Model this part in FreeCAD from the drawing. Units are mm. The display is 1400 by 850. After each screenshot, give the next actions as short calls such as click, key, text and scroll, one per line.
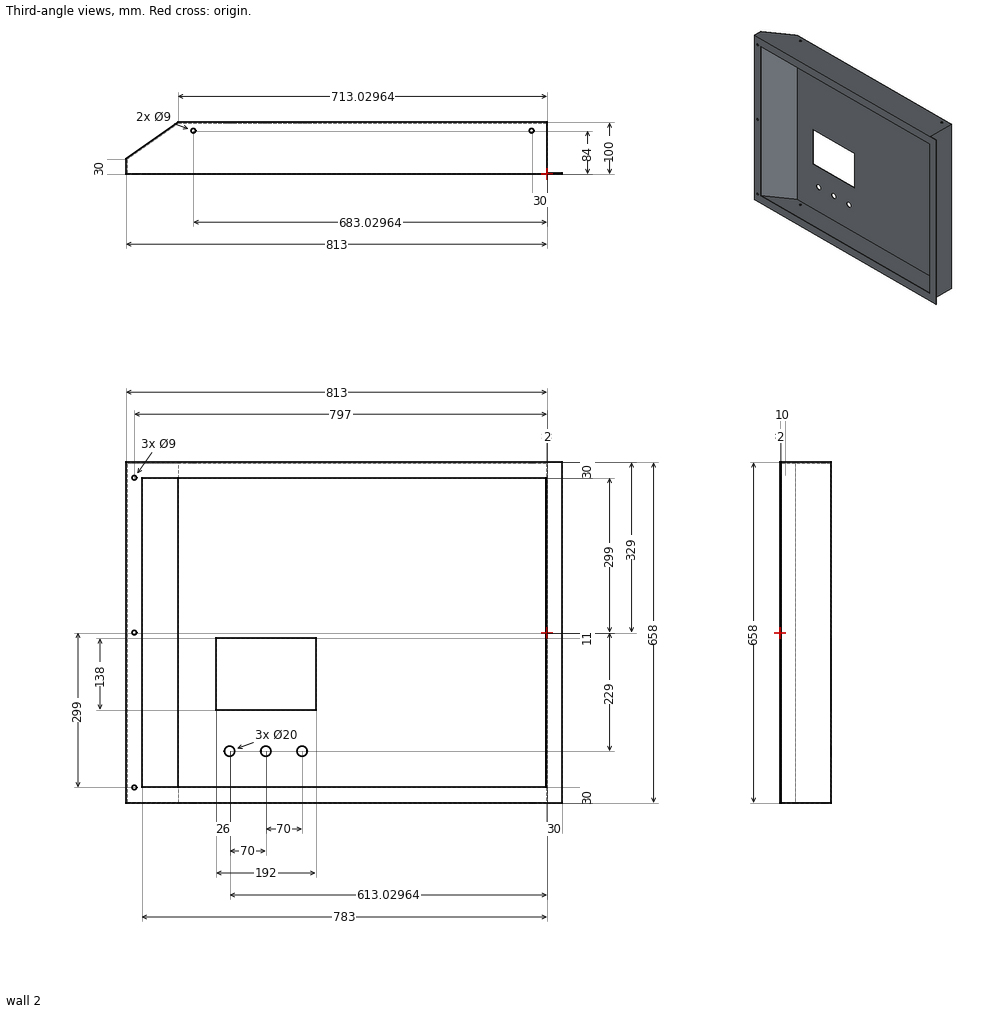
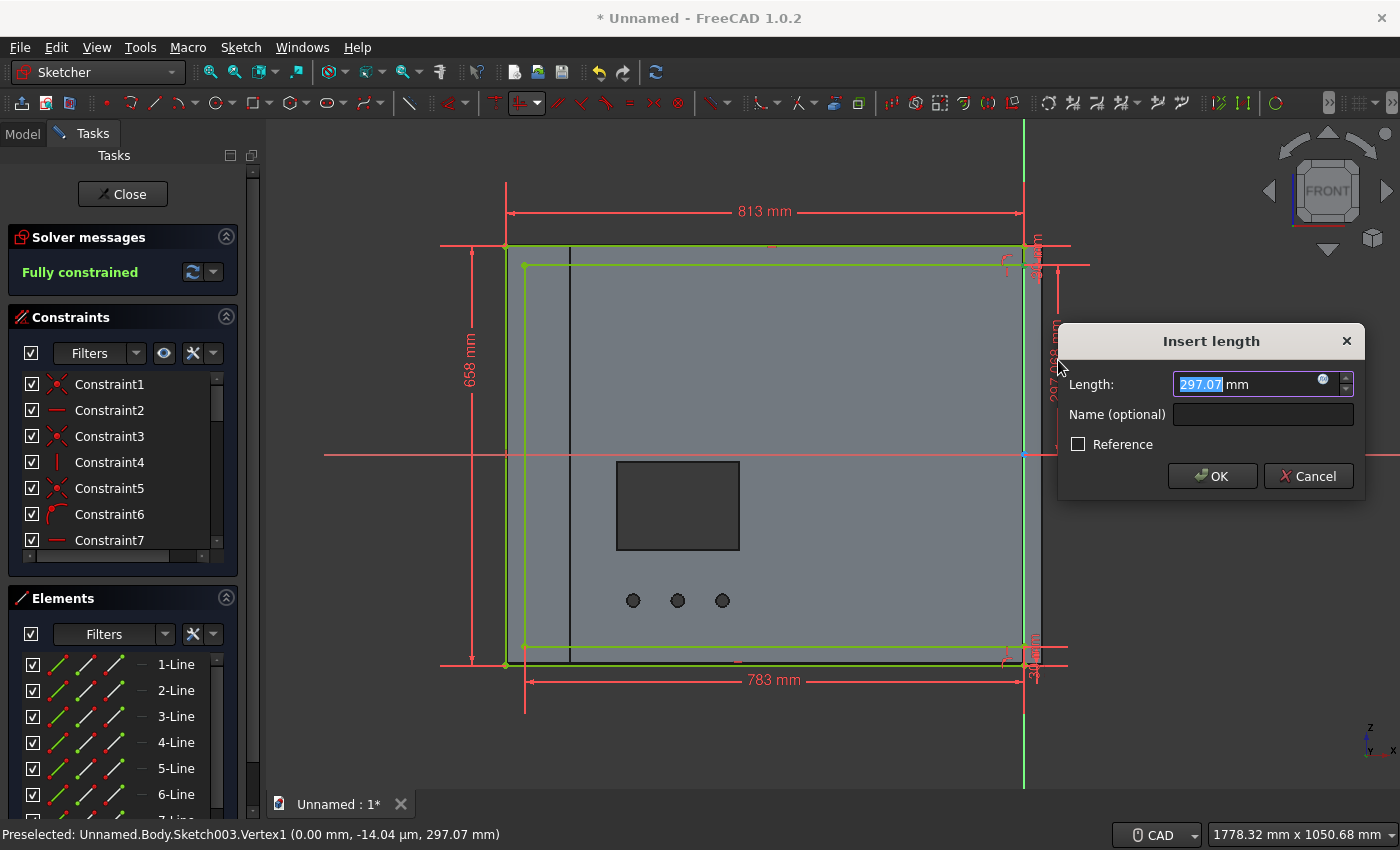
text(299)
key(Return)
key(Escape)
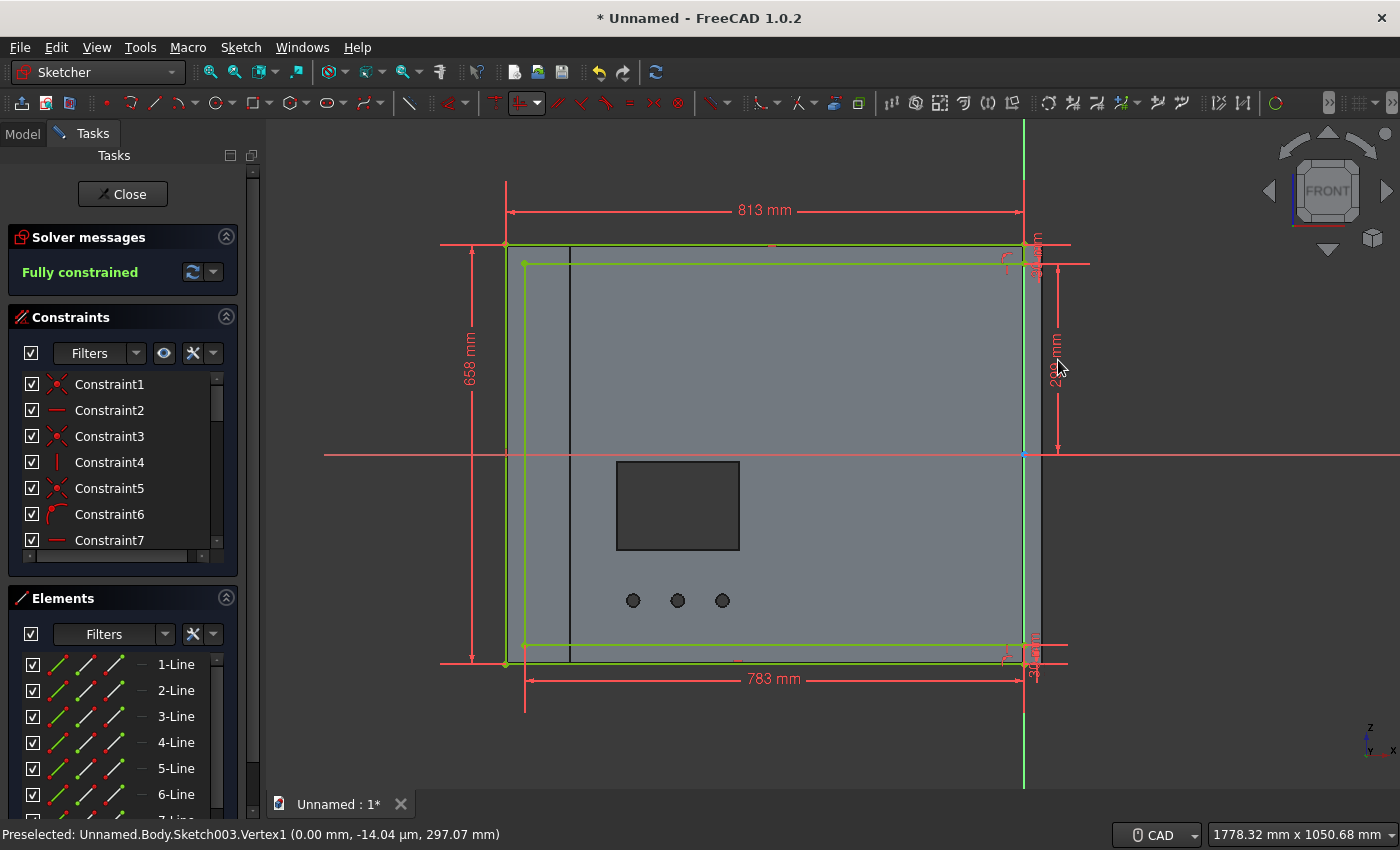
click(123, 194)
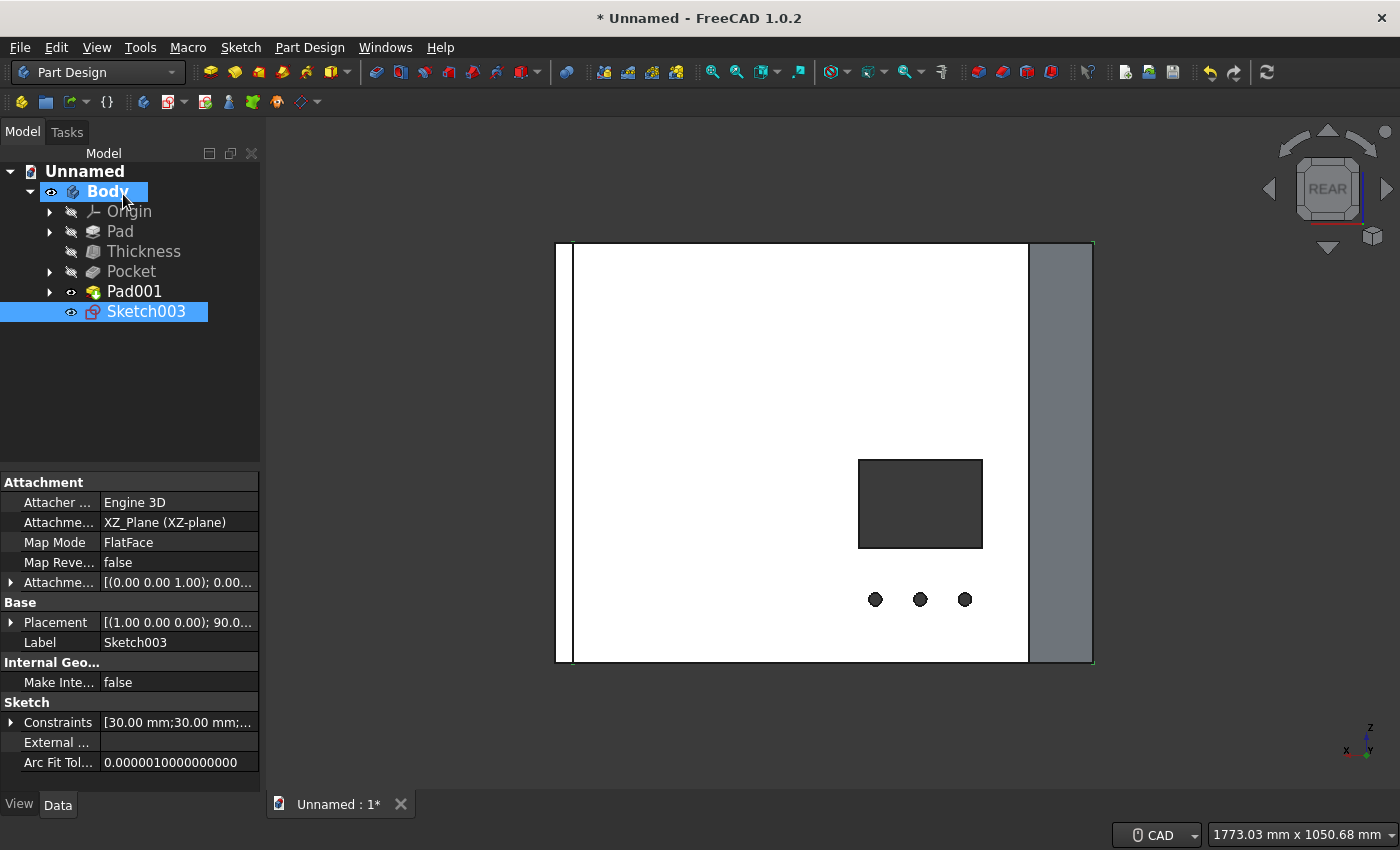
click(212, 72)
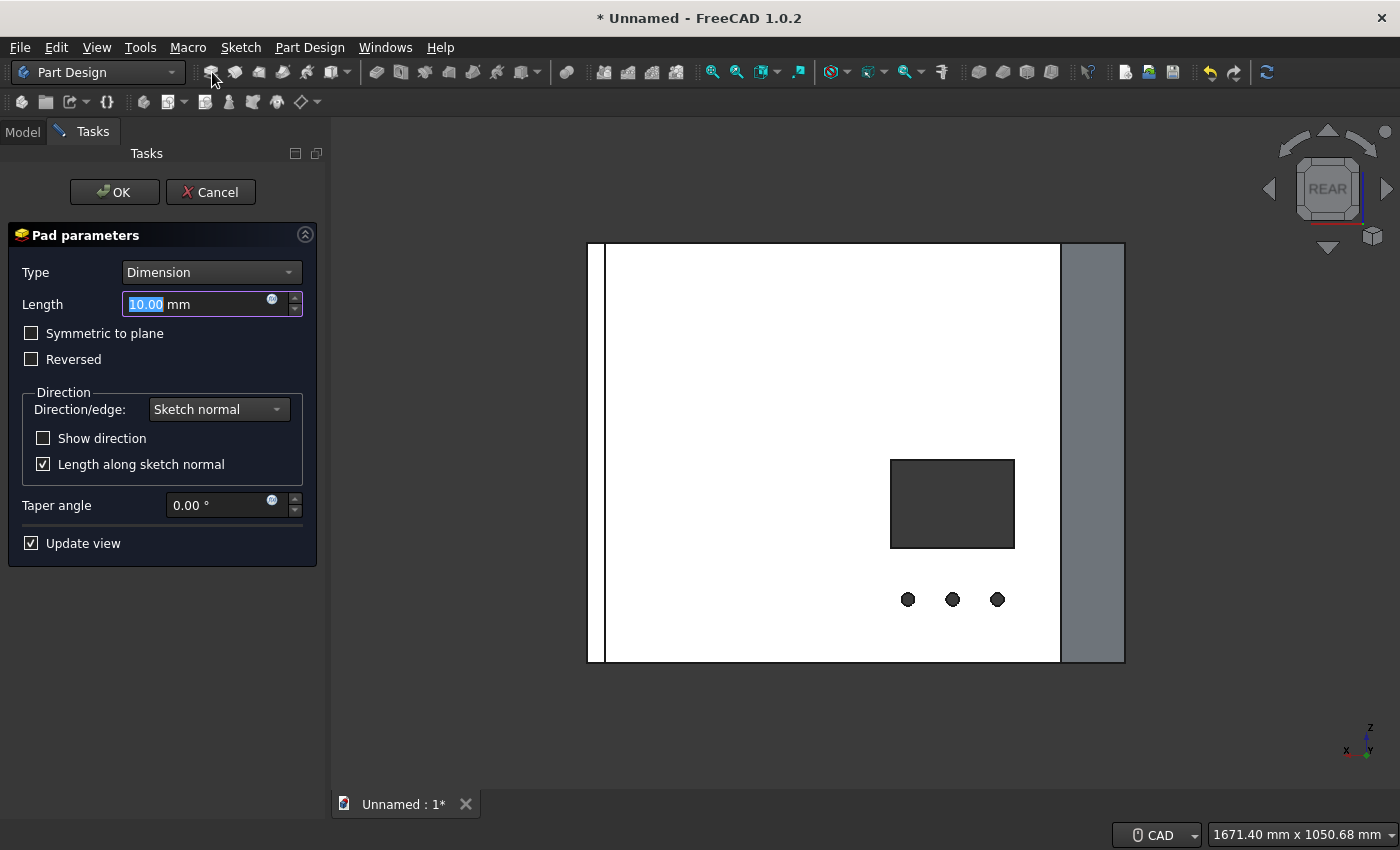
text(2)
key(Tab)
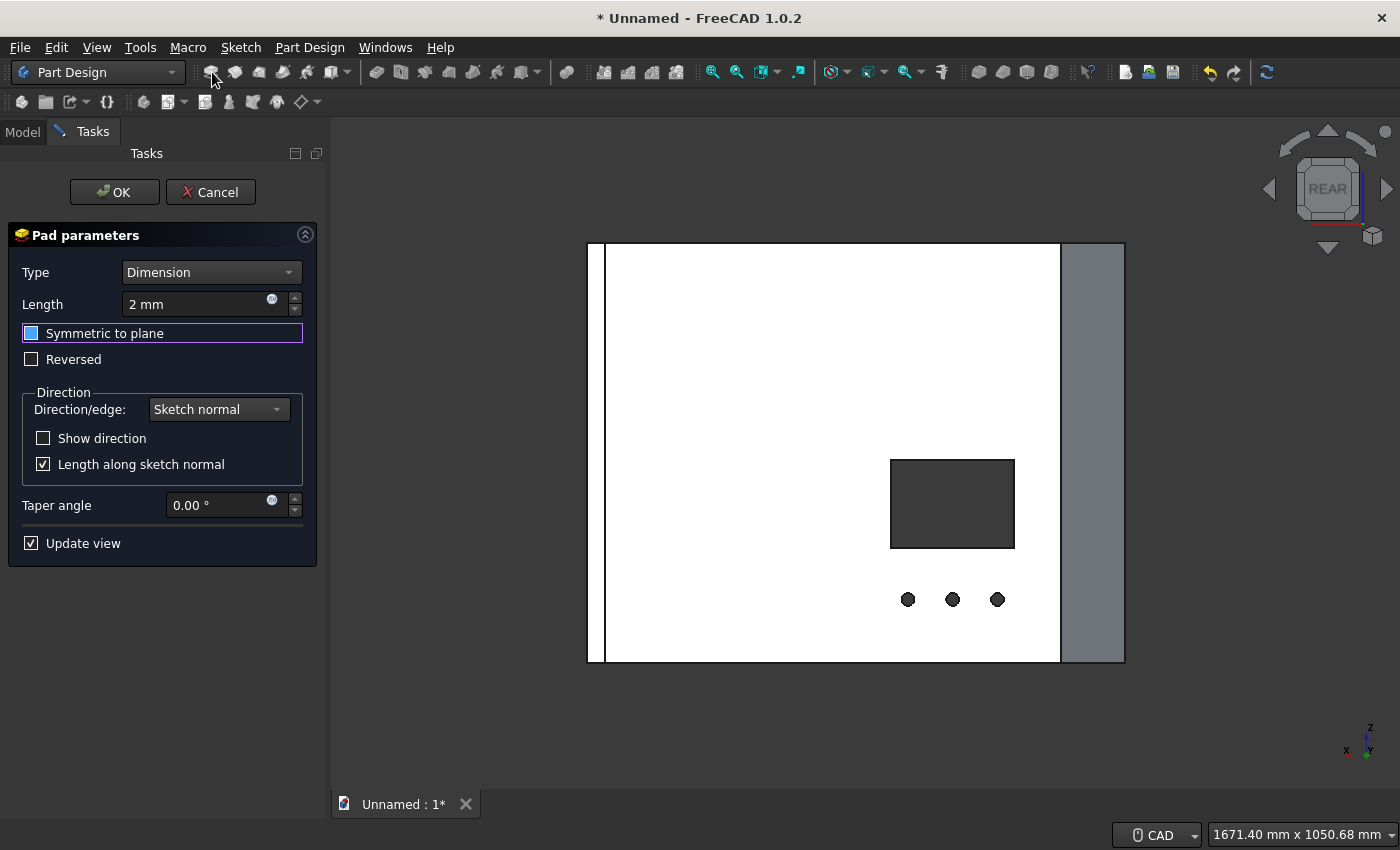
click(30, 359)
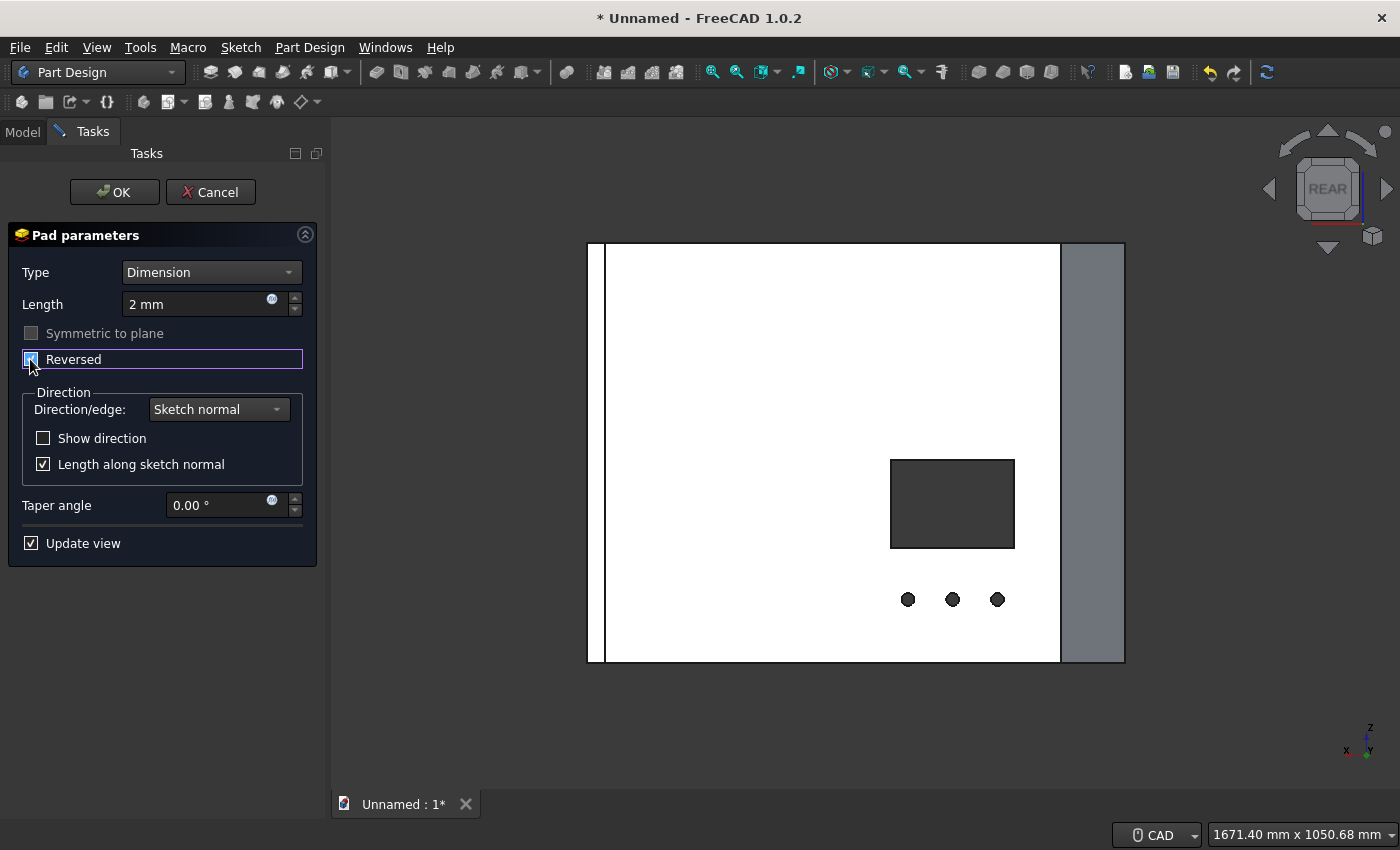
click(115, 192)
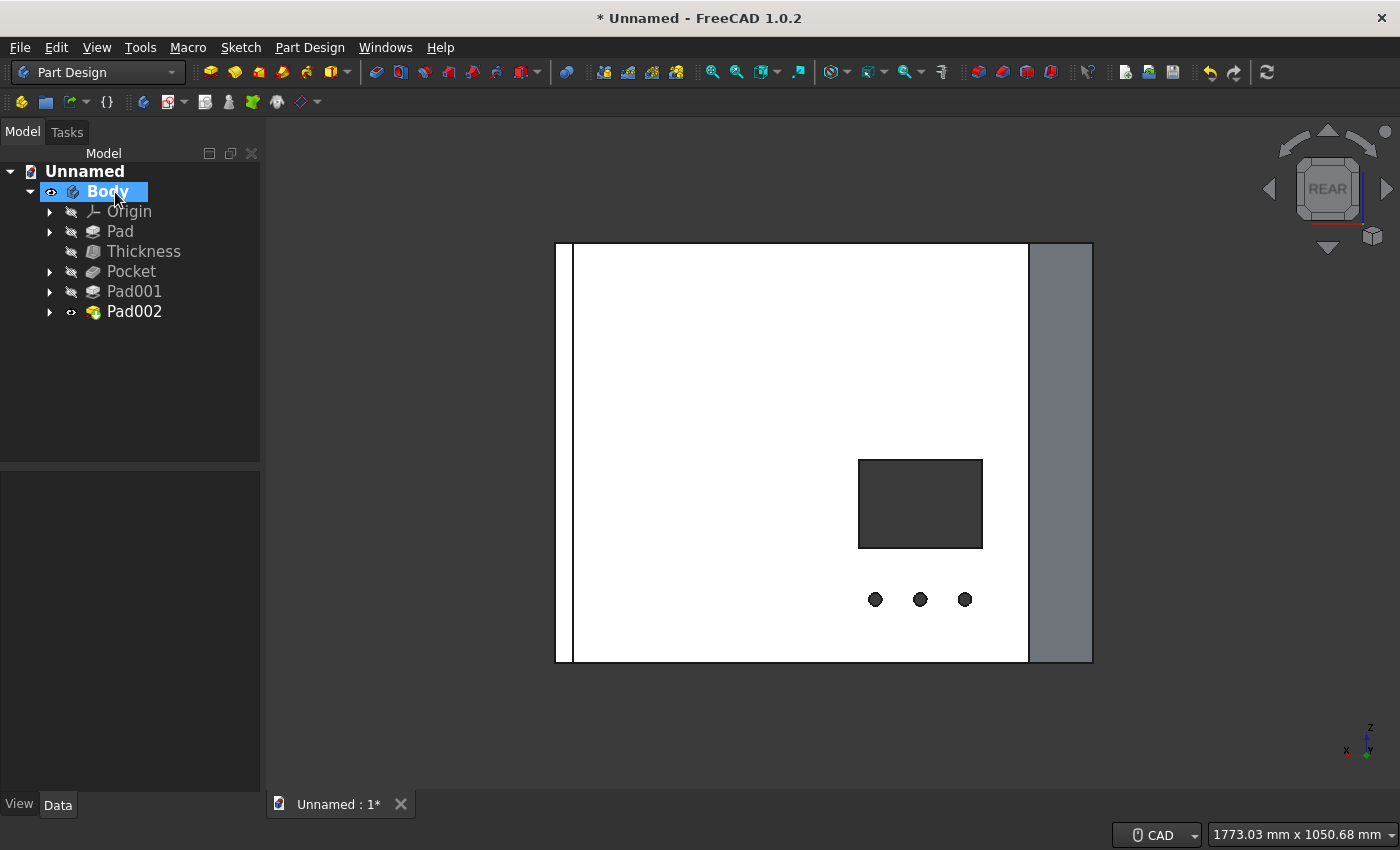
key(0)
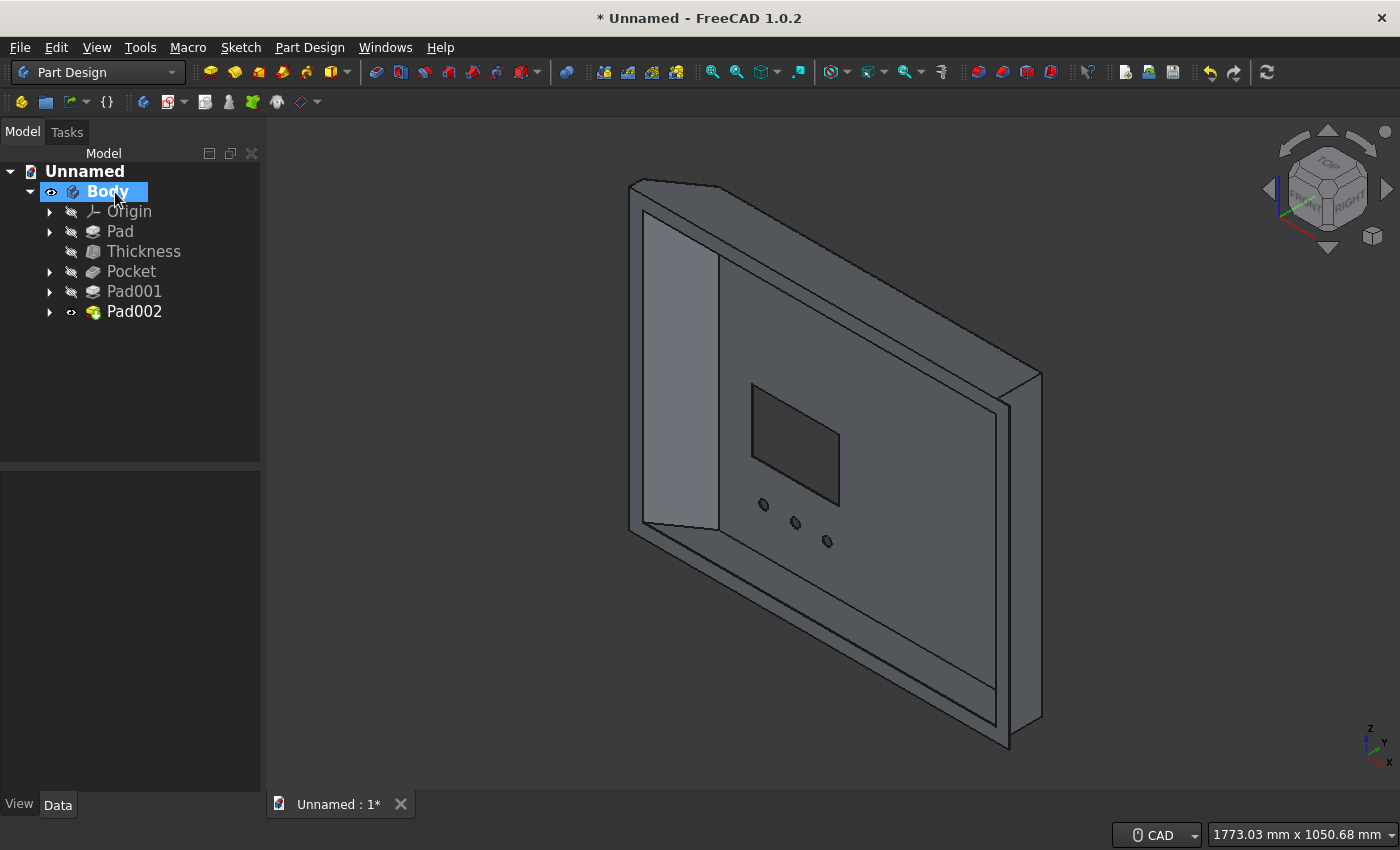
click(950, 345)